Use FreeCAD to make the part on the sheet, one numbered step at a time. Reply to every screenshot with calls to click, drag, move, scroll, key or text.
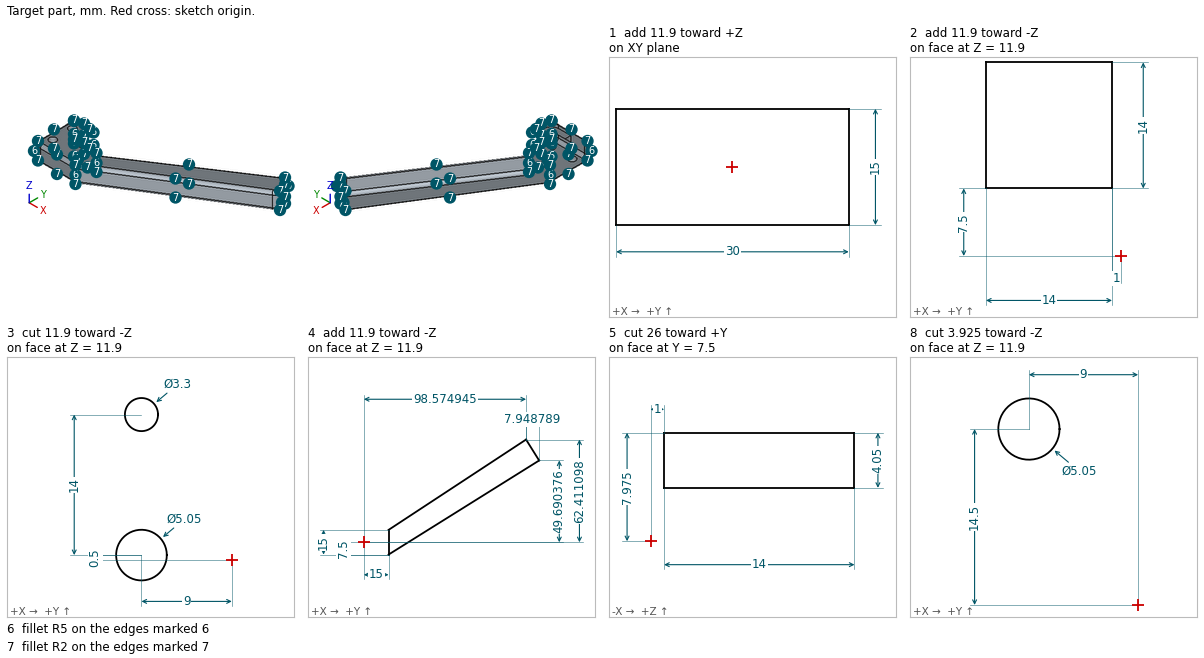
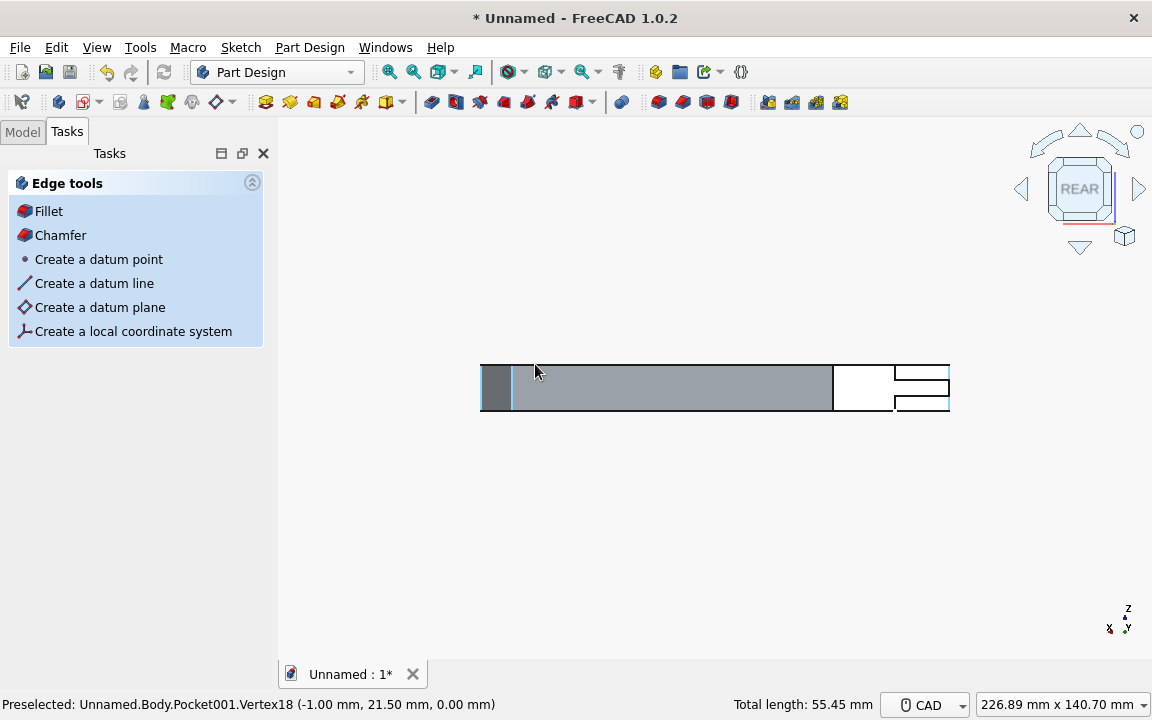
click(895, 402, ctrl)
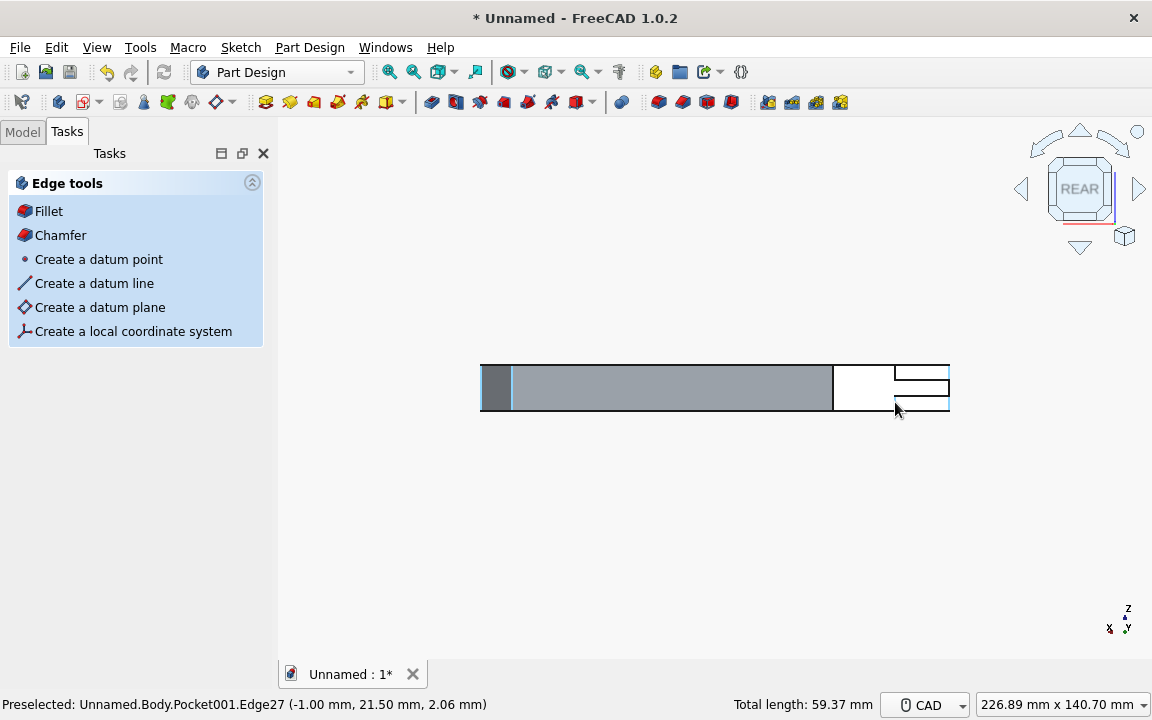
click(895, 372, ctrl)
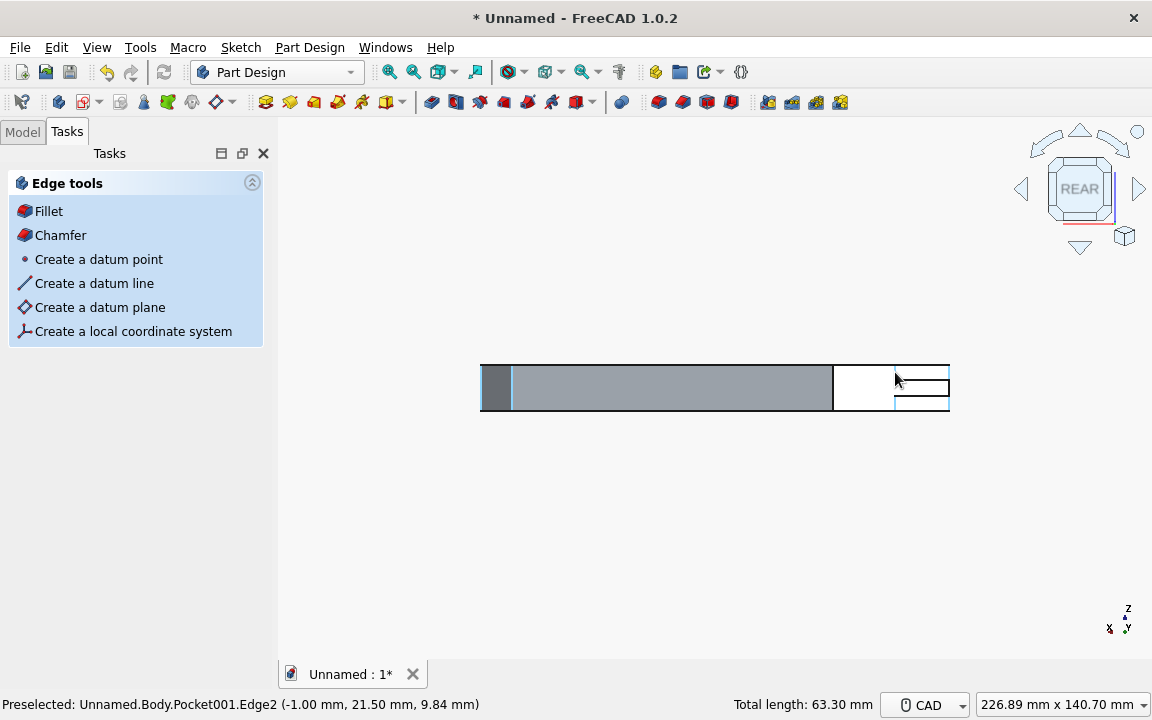
scroll(895, 402, up, 5)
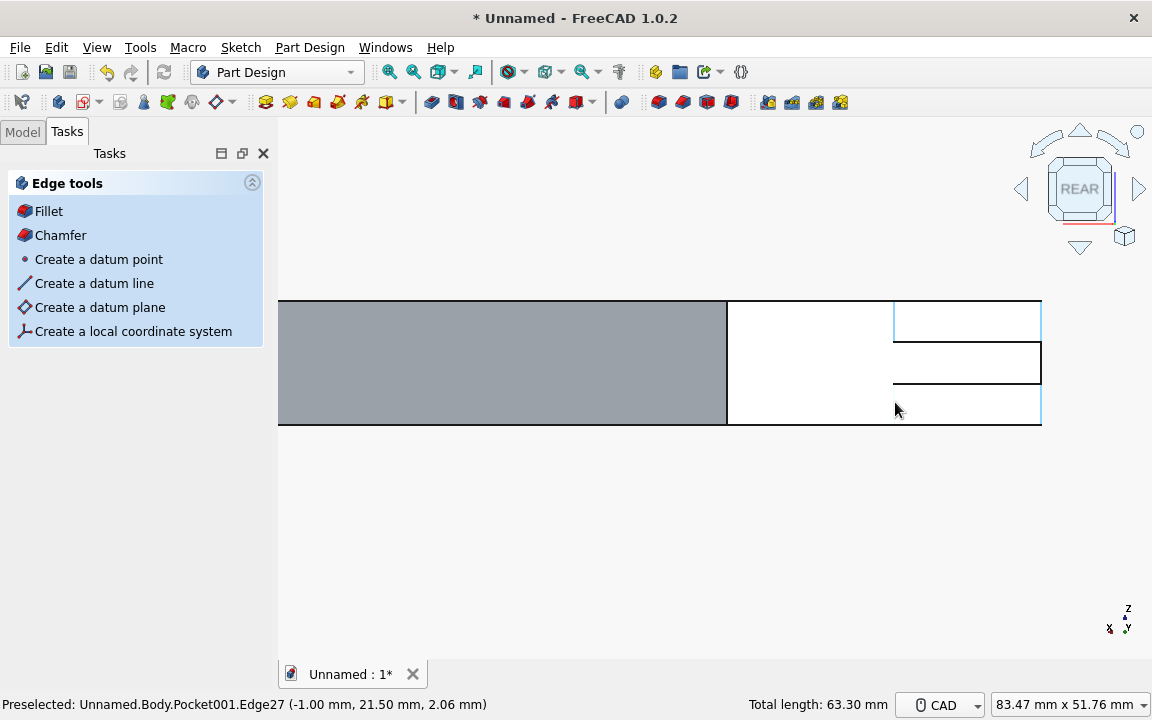
click(390, 72)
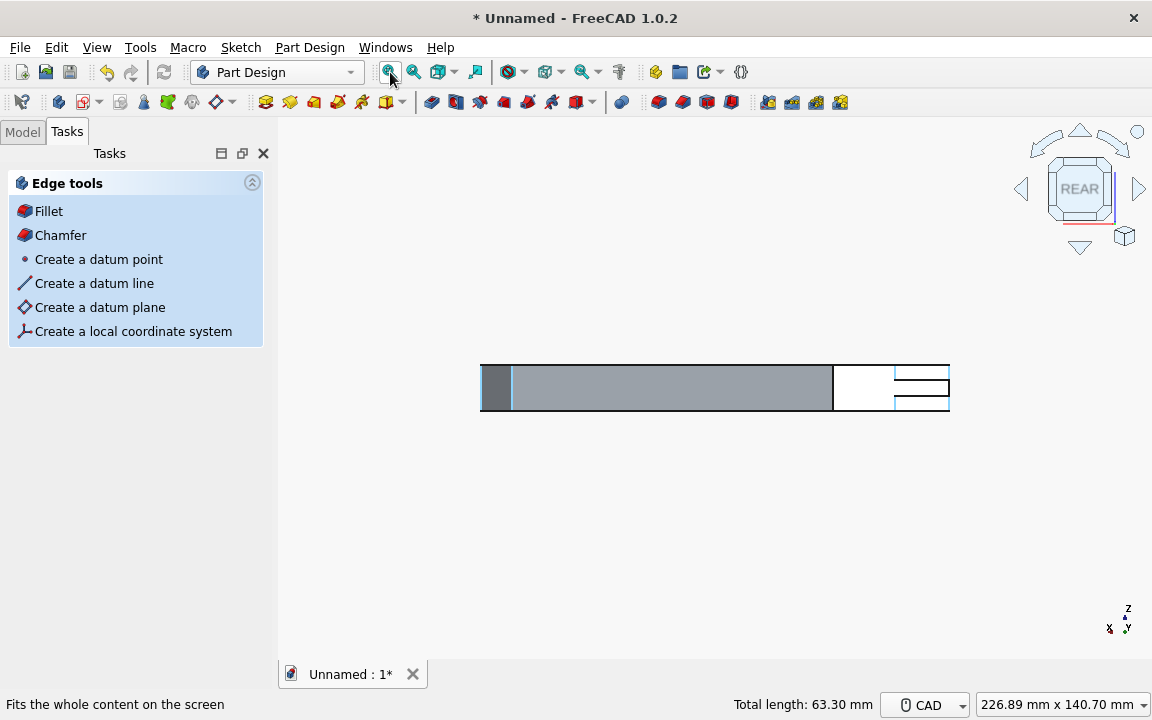
key(6)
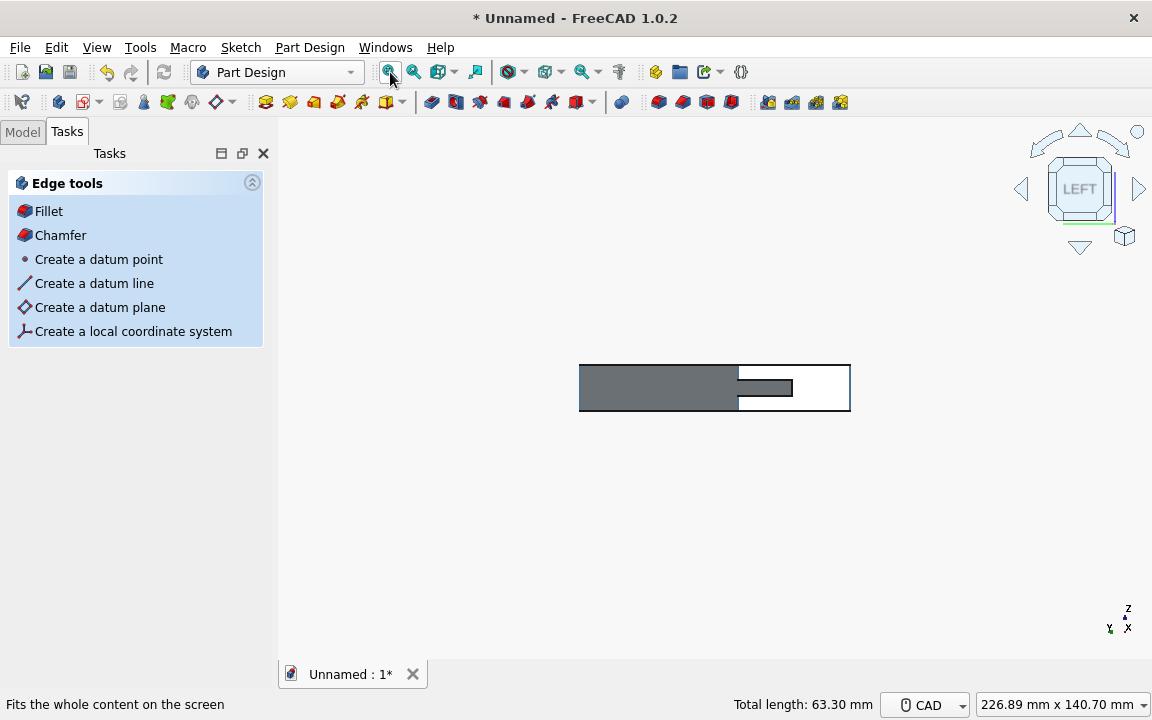
click(390, 72)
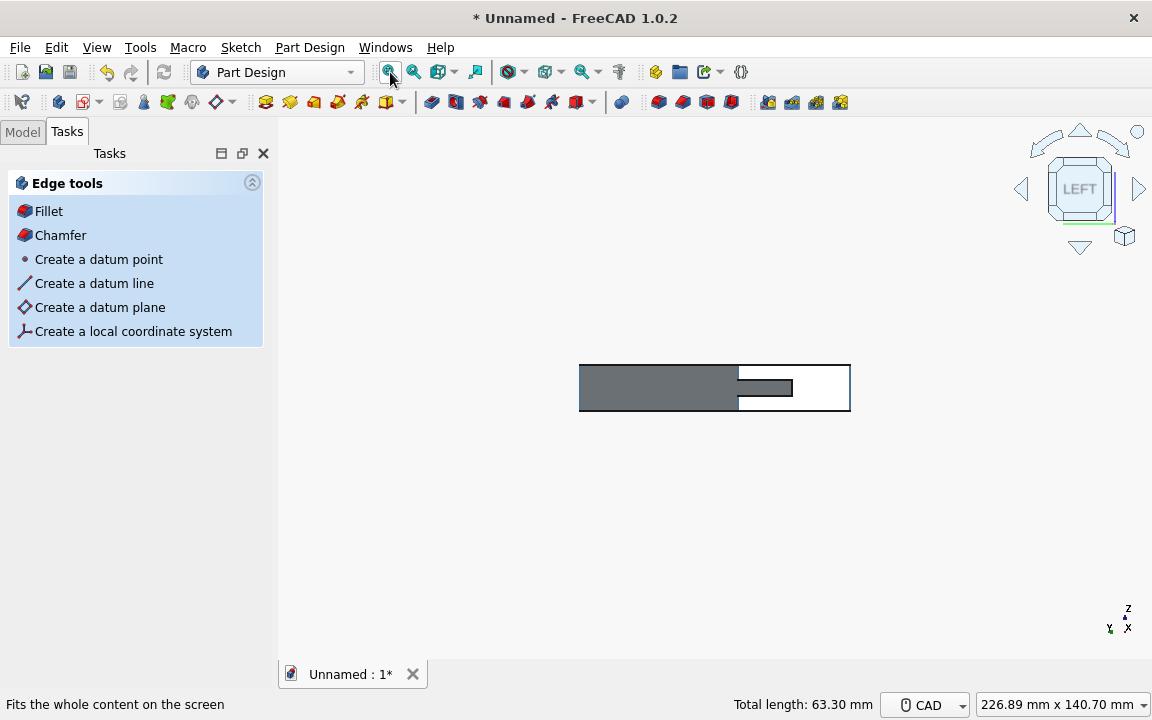
scroll(792, 402, up, 5)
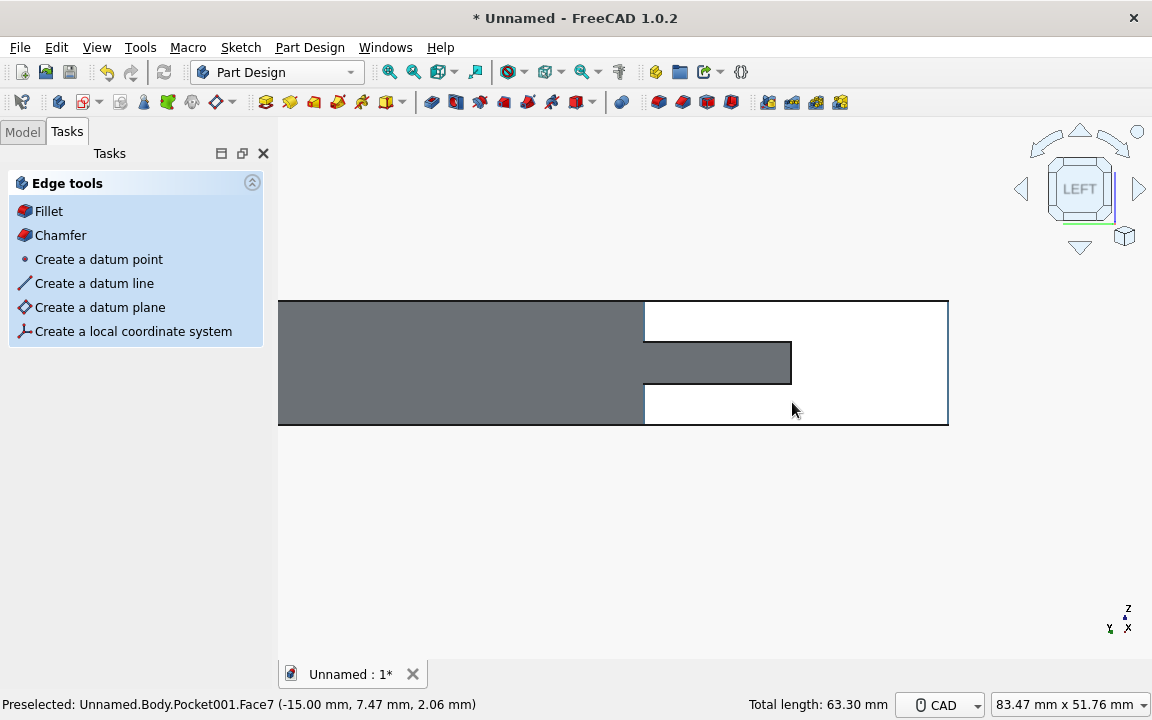
click(390, 72)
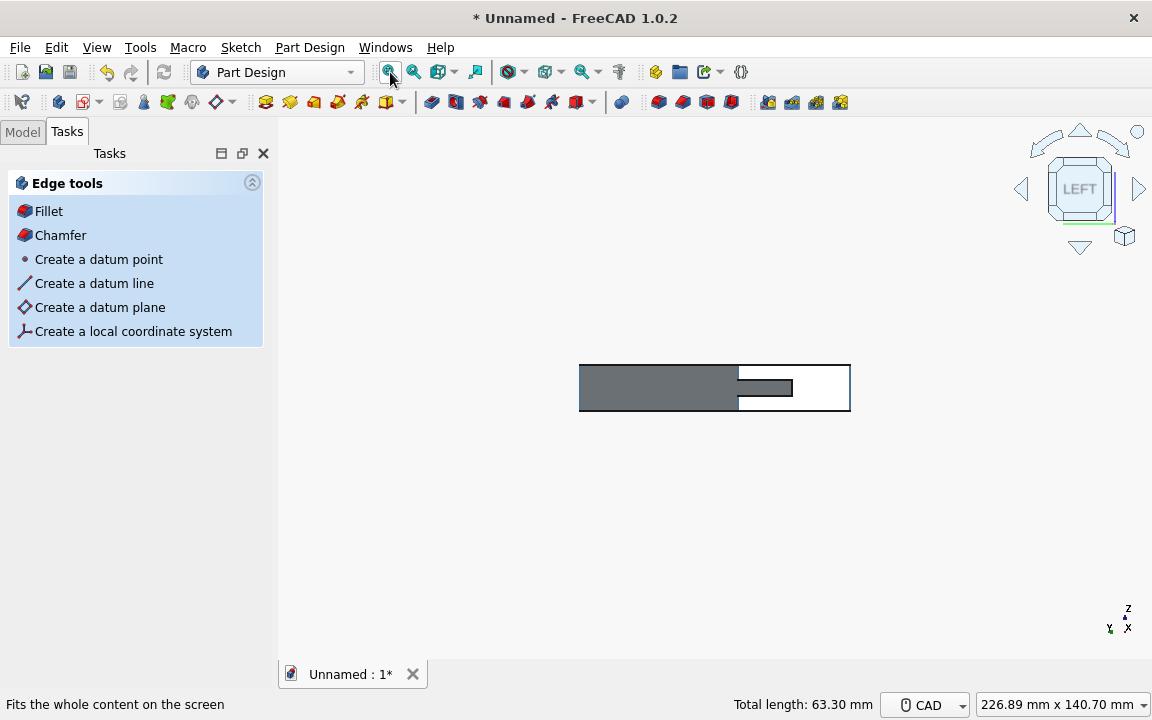
key(v)
key(3)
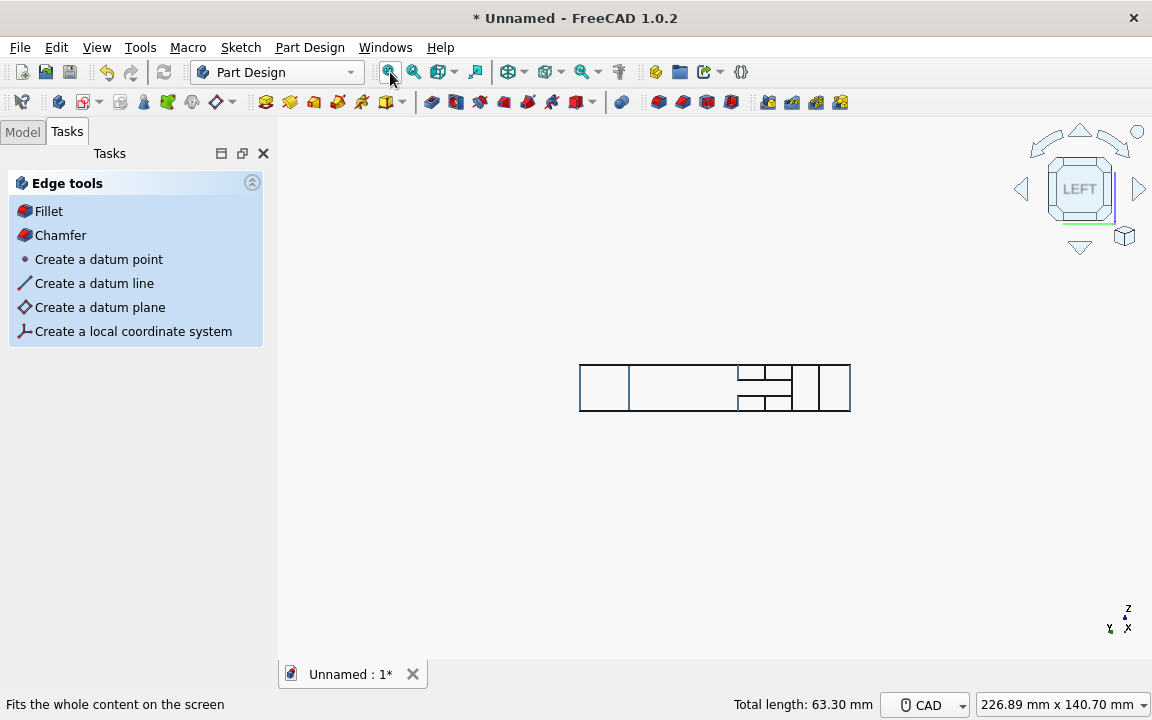
key(0)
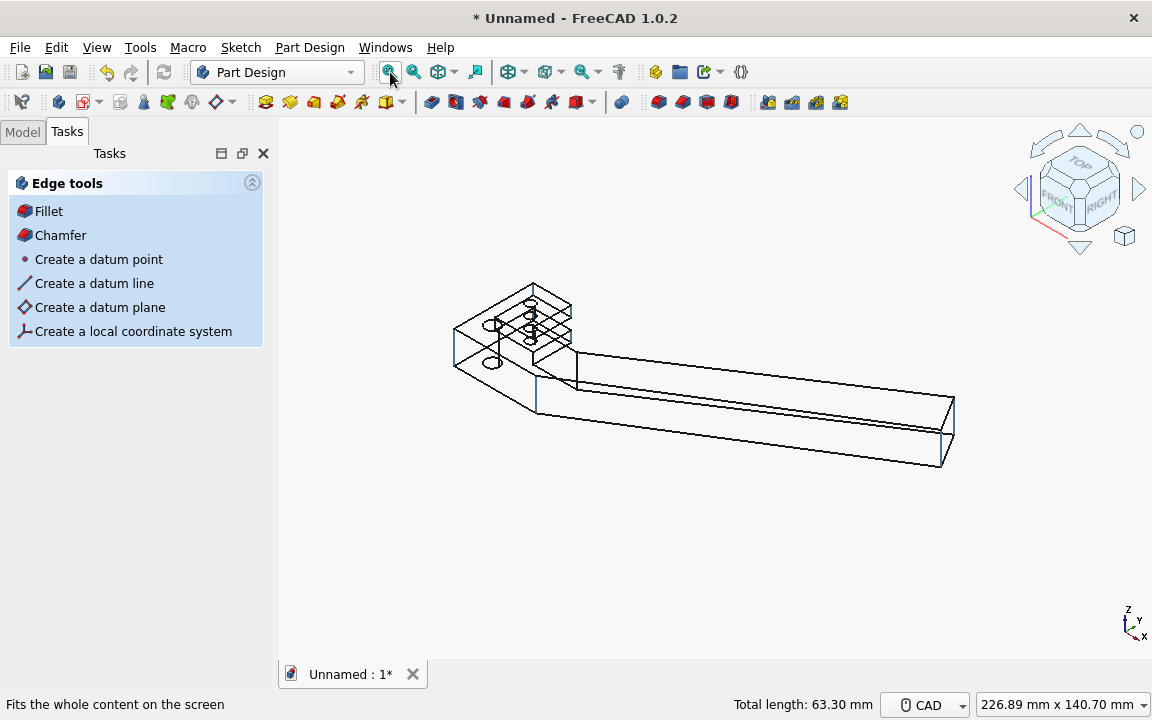
click(533, 359, ctrl)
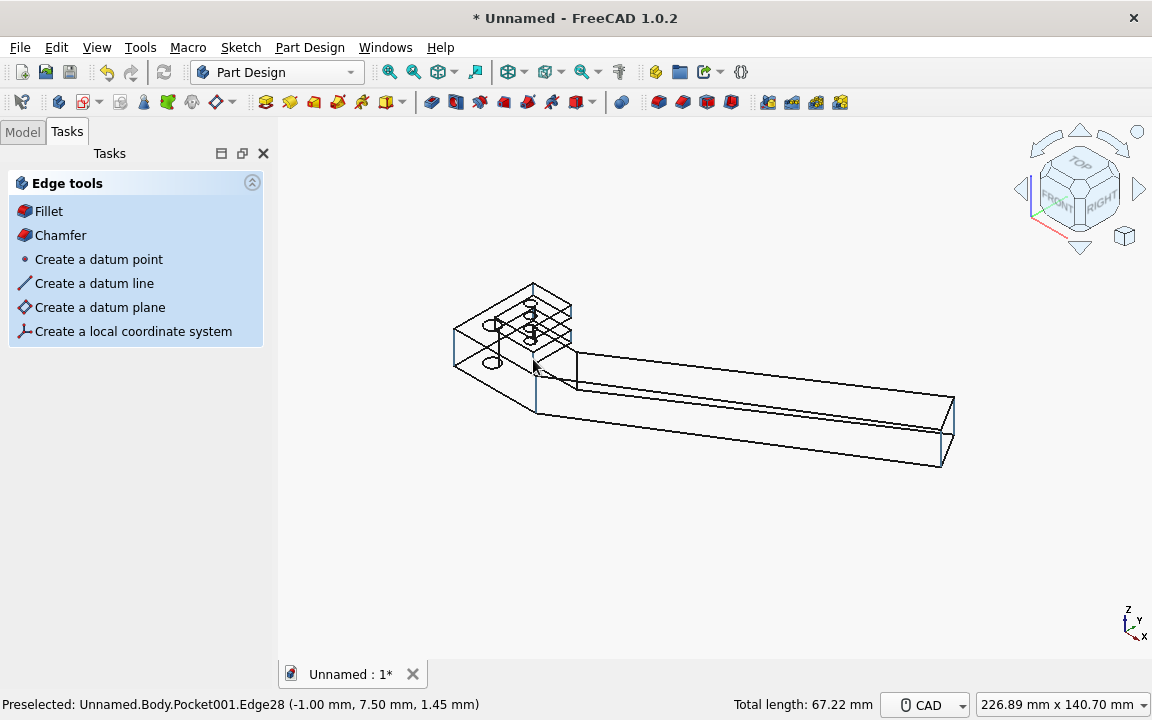
click(533, 334, ctrl)